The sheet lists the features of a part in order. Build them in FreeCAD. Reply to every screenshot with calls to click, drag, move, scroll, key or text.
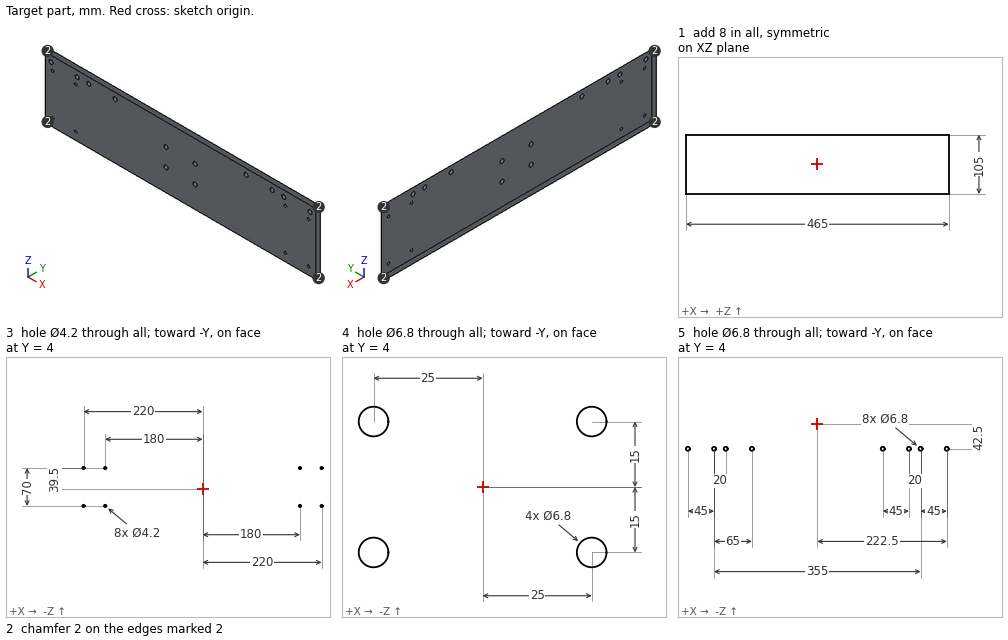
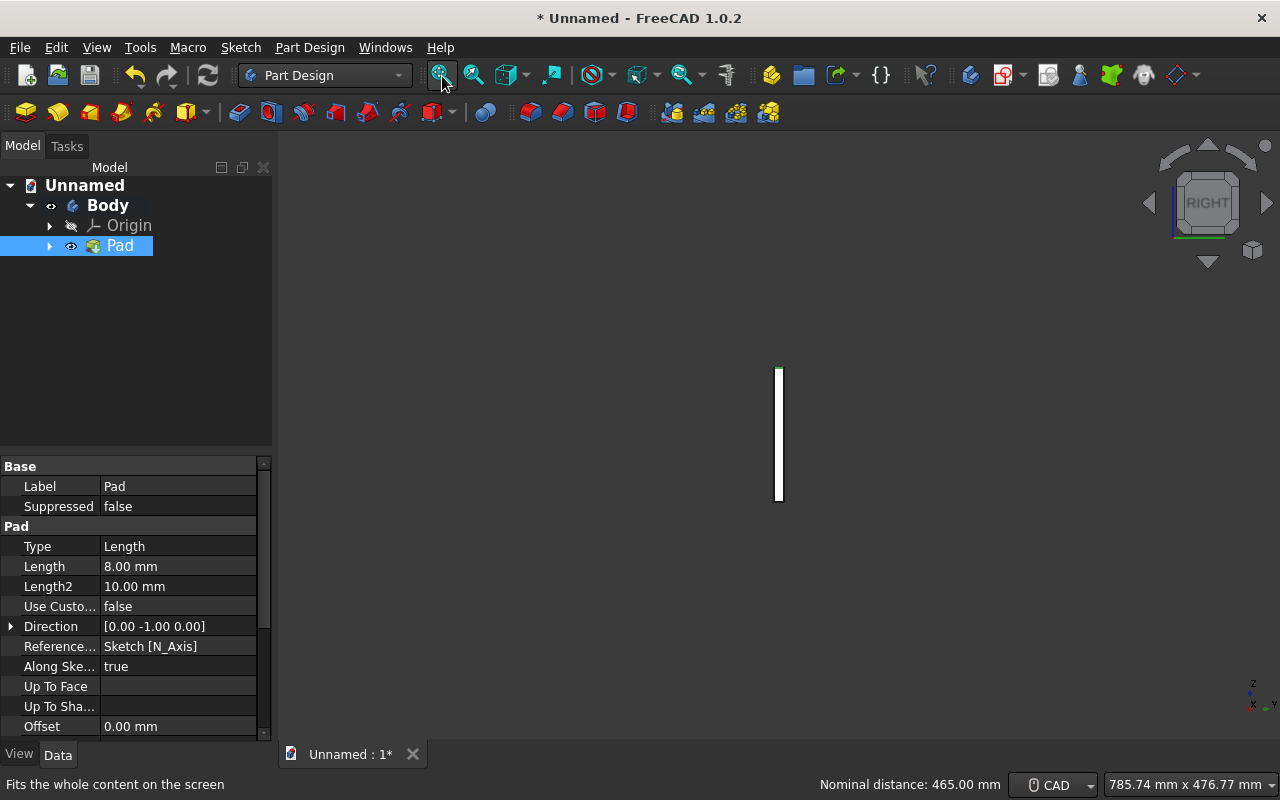
scroll(779, 501, up, 7)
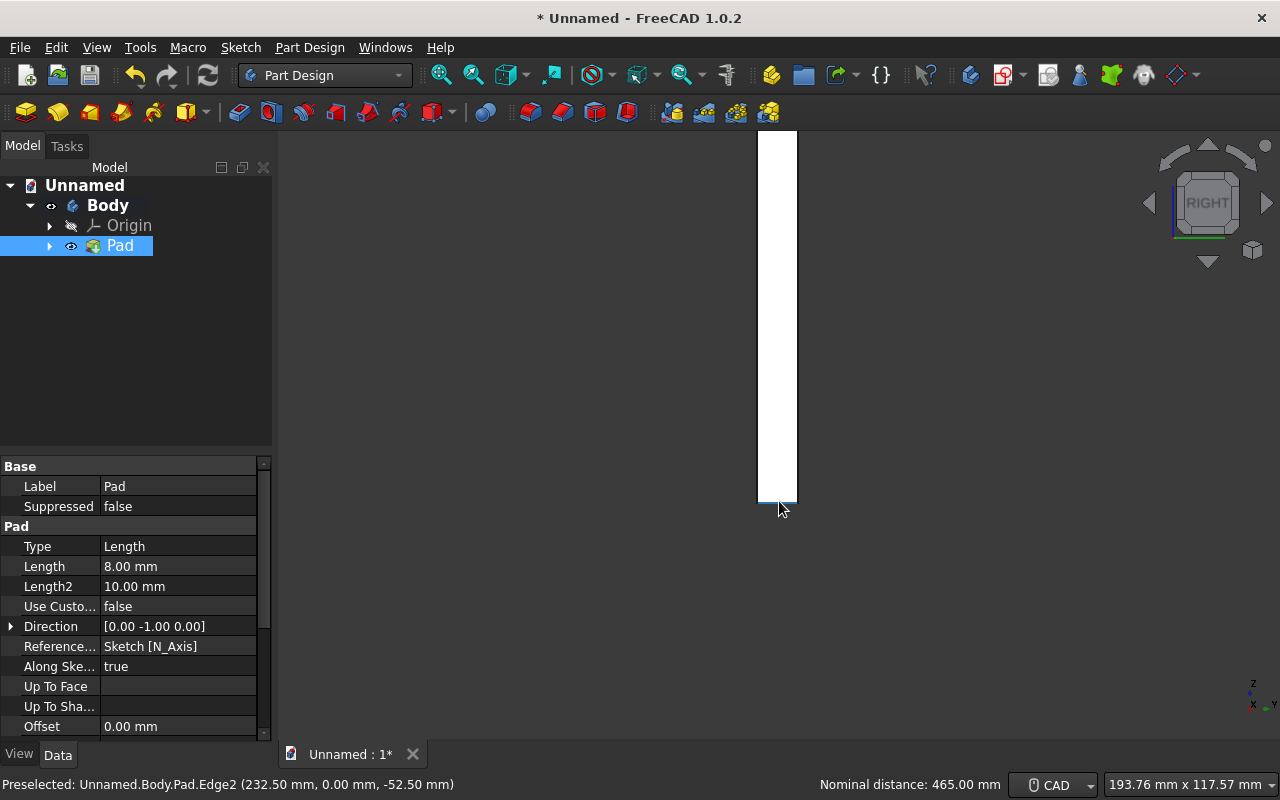
click(777, 502, ctrl)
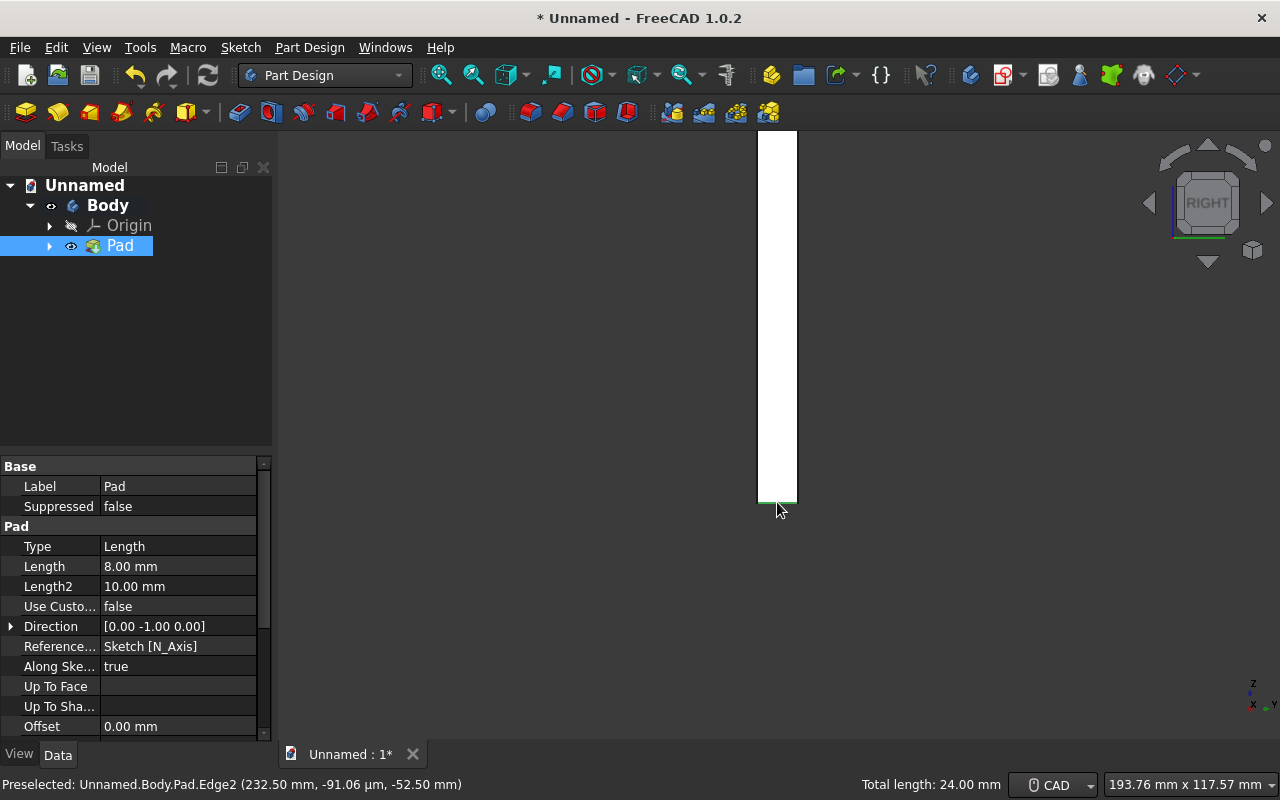
click(442, 76)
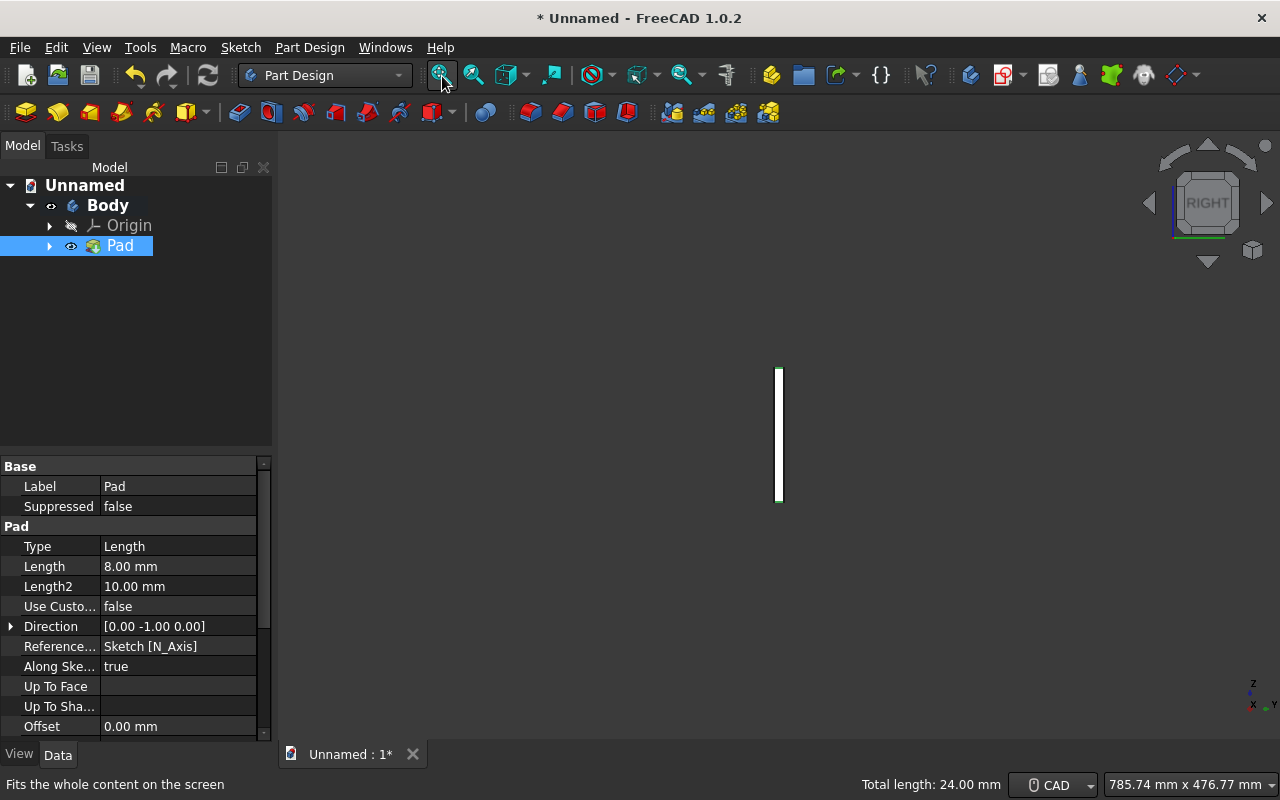
key(5)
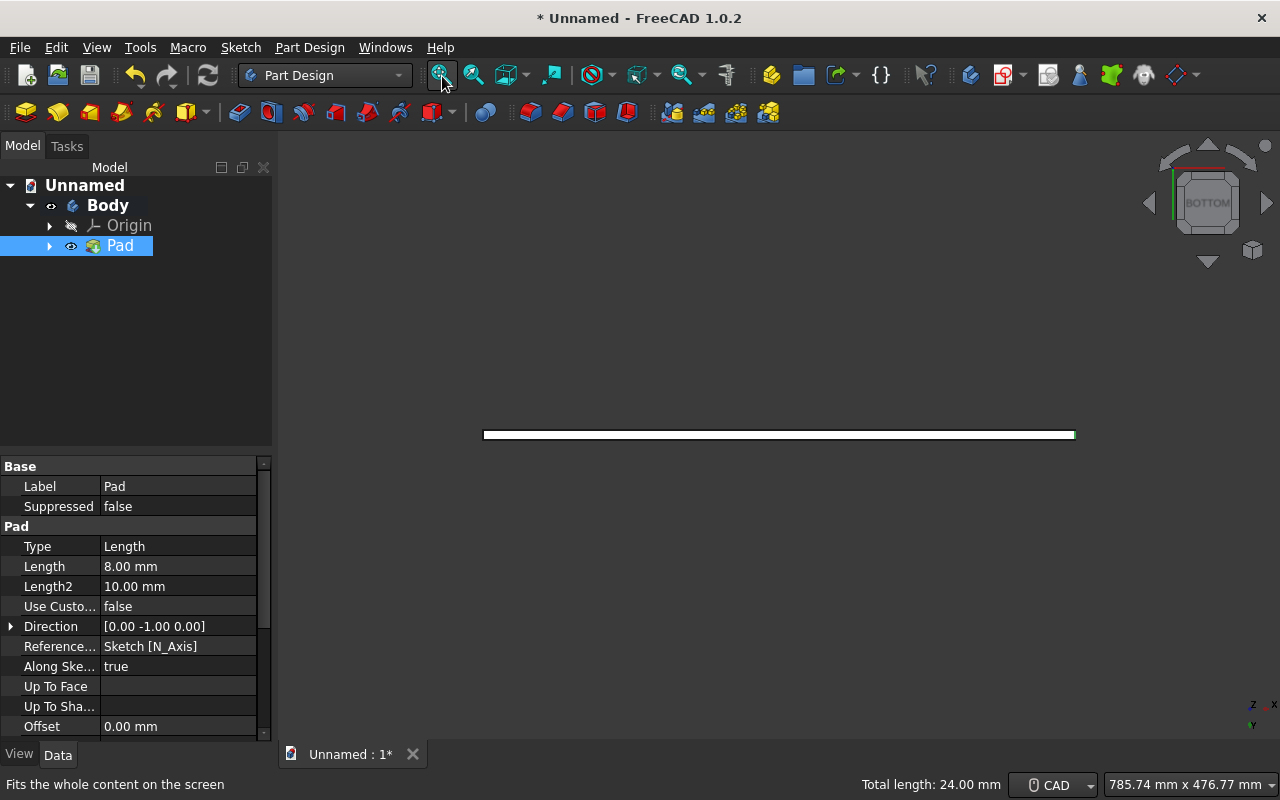
click(483, 435, ctrl)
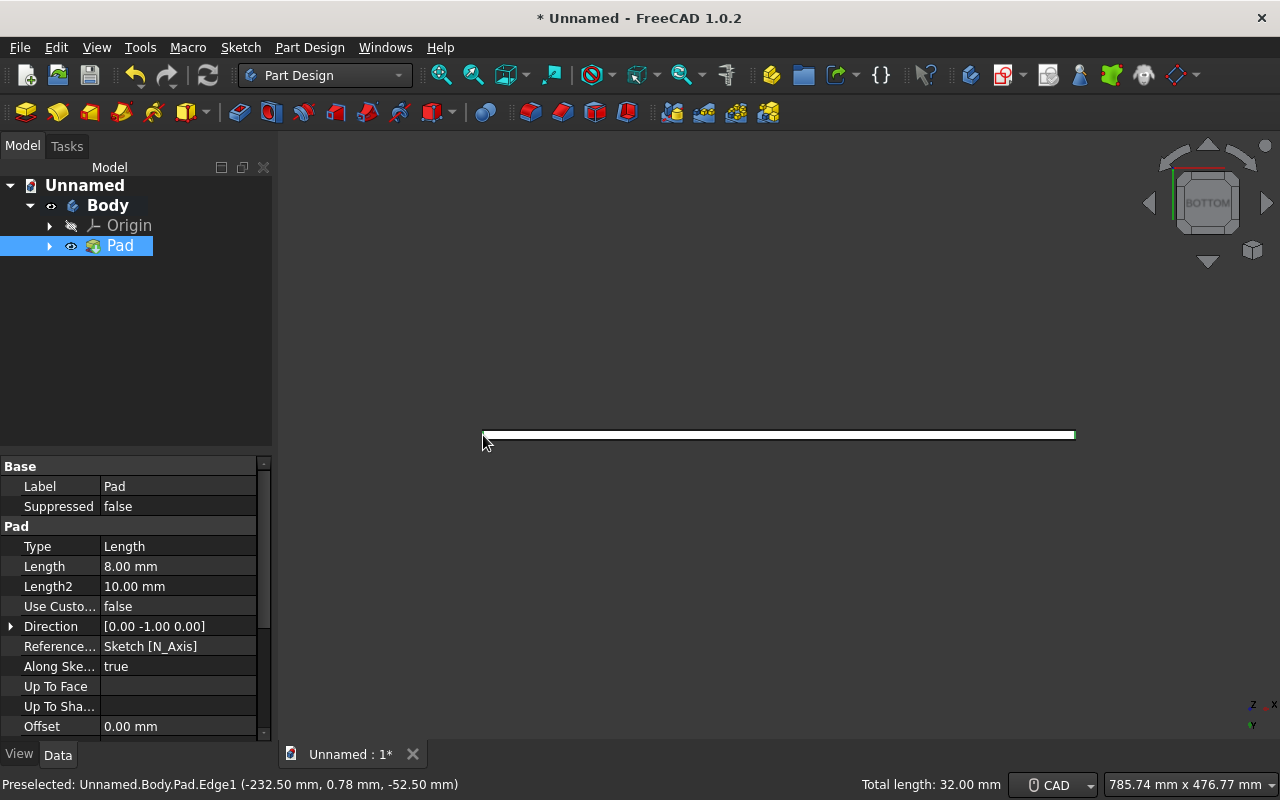
click(564, 112)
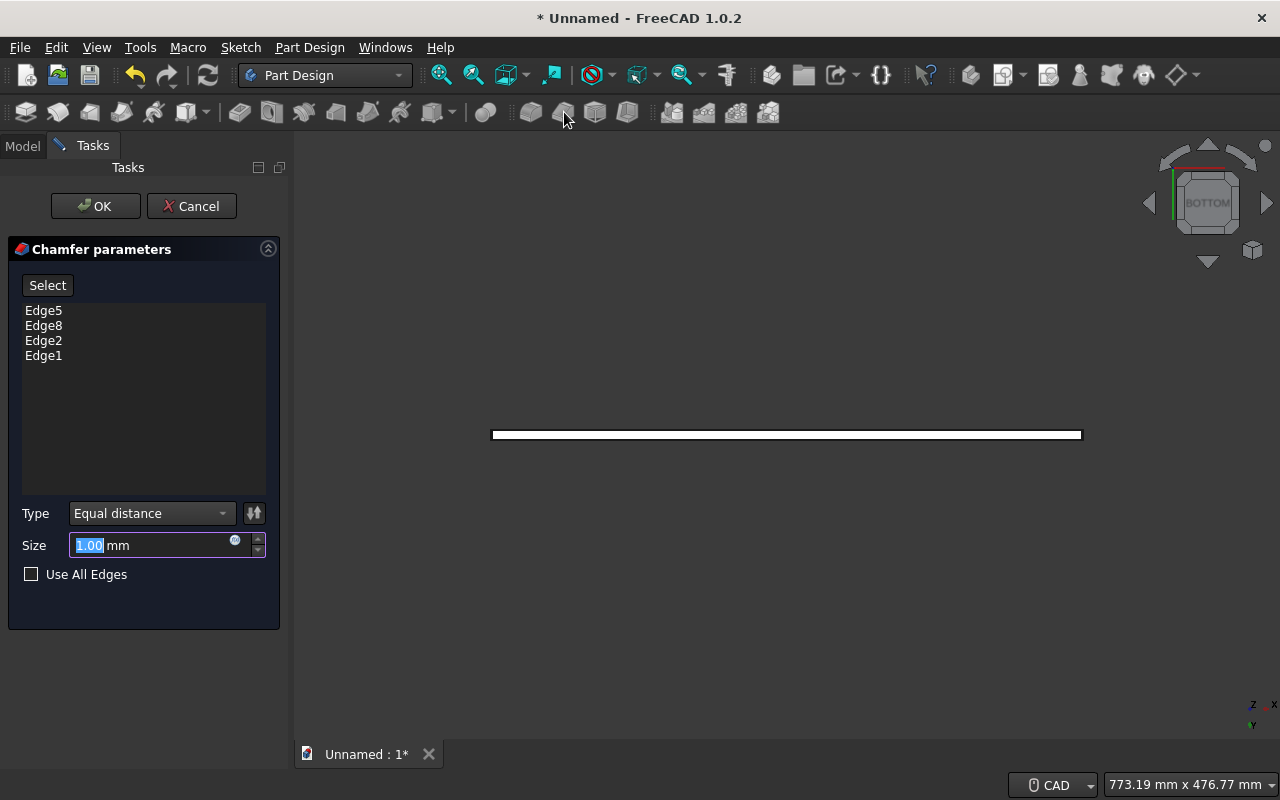
text(2)
key(Tab)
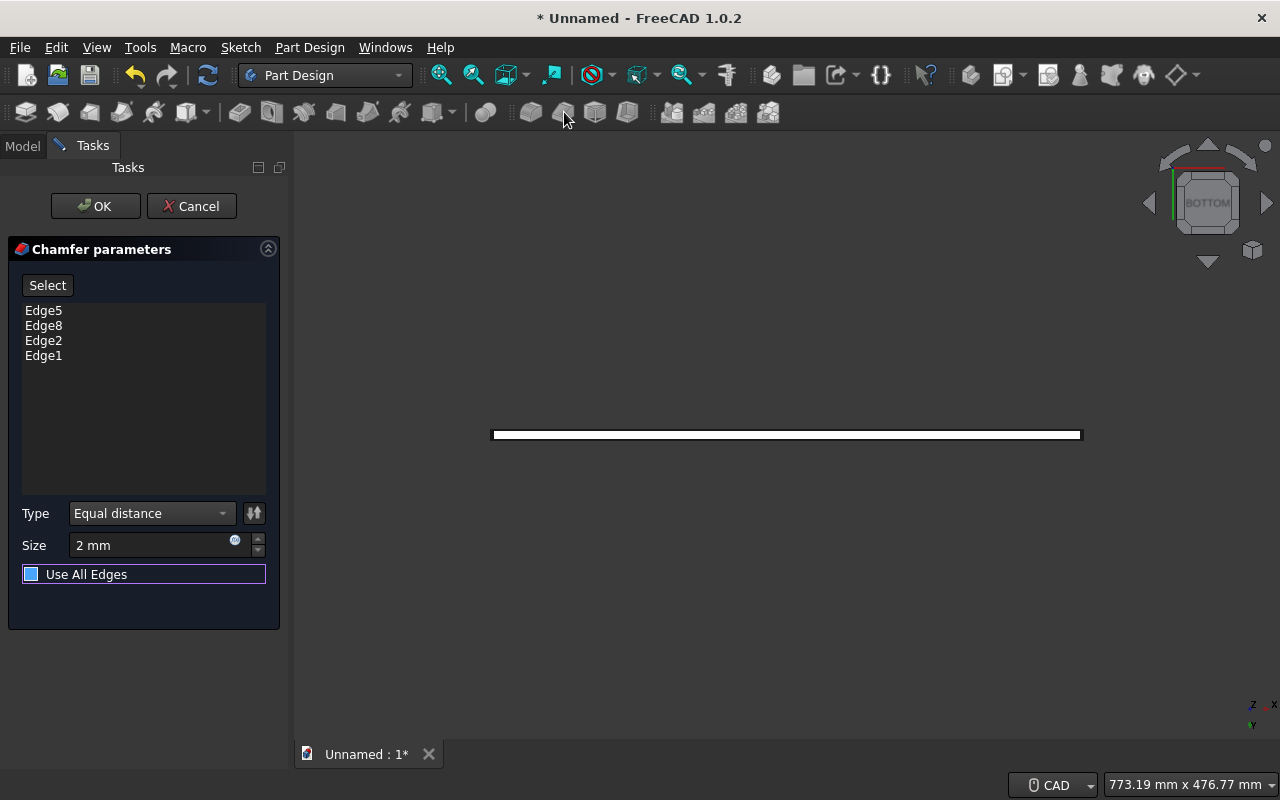
click(96, 206)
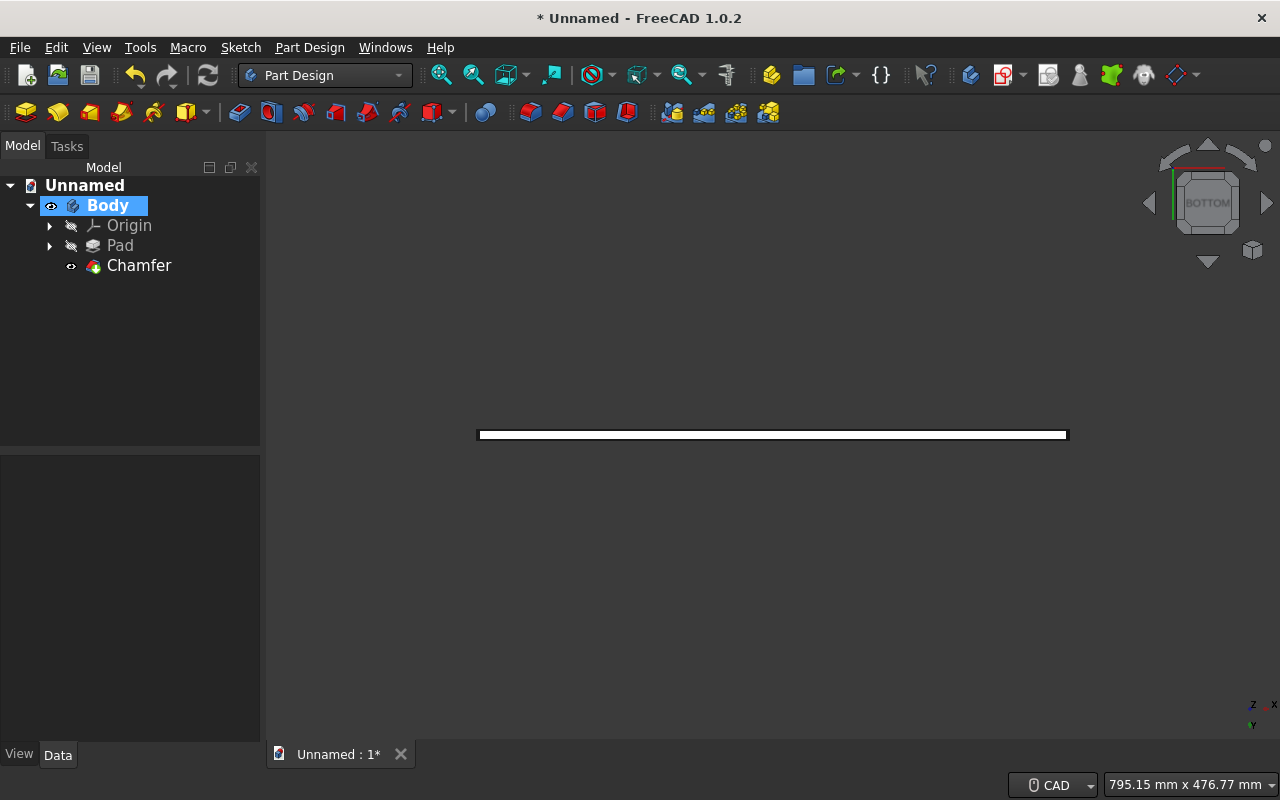
key(4)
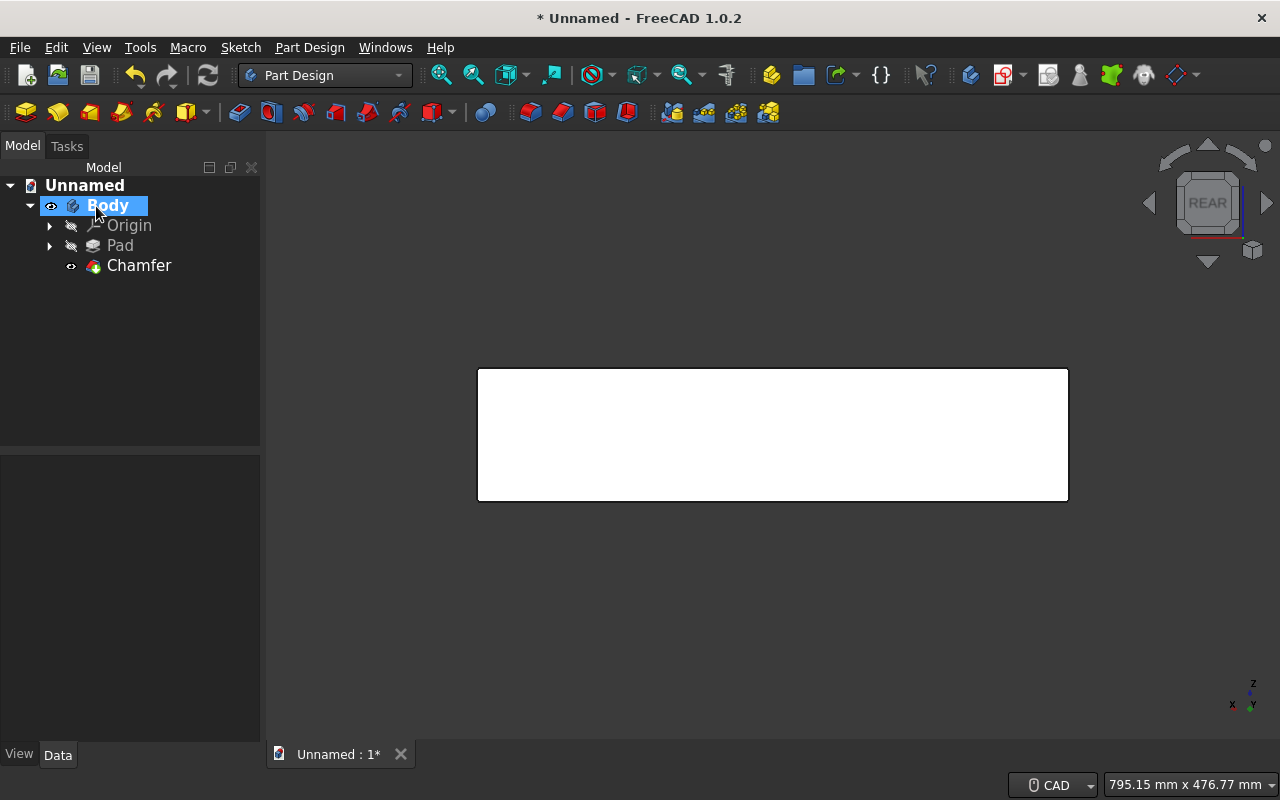
click(604, 434)